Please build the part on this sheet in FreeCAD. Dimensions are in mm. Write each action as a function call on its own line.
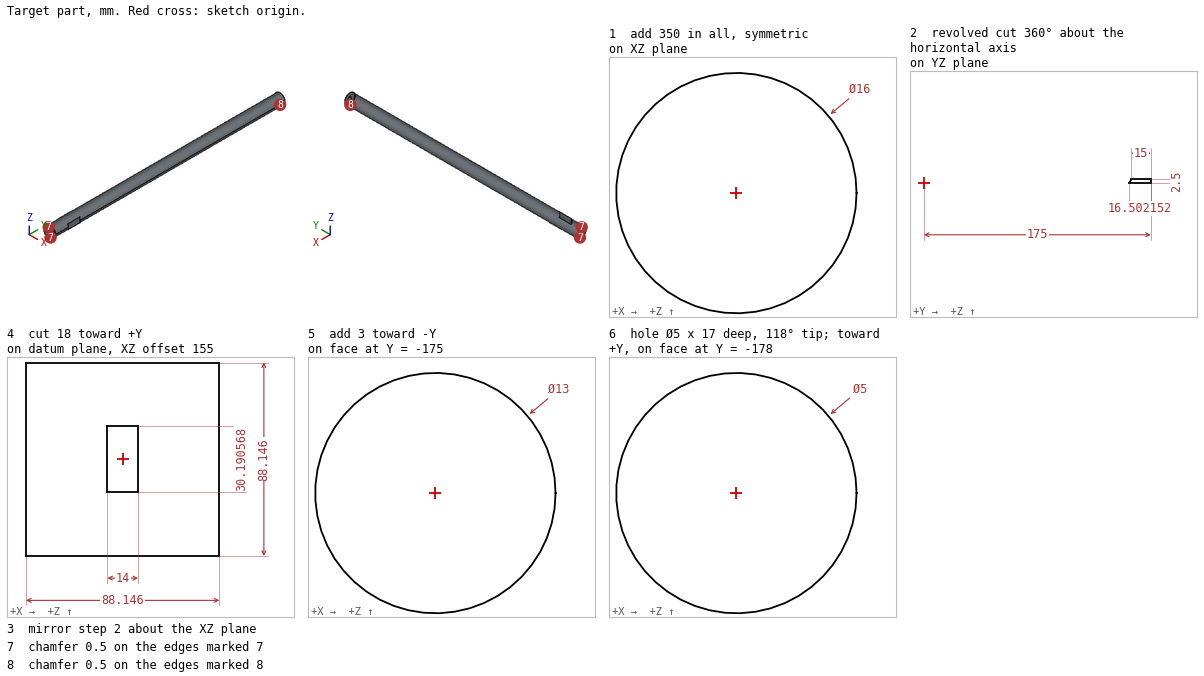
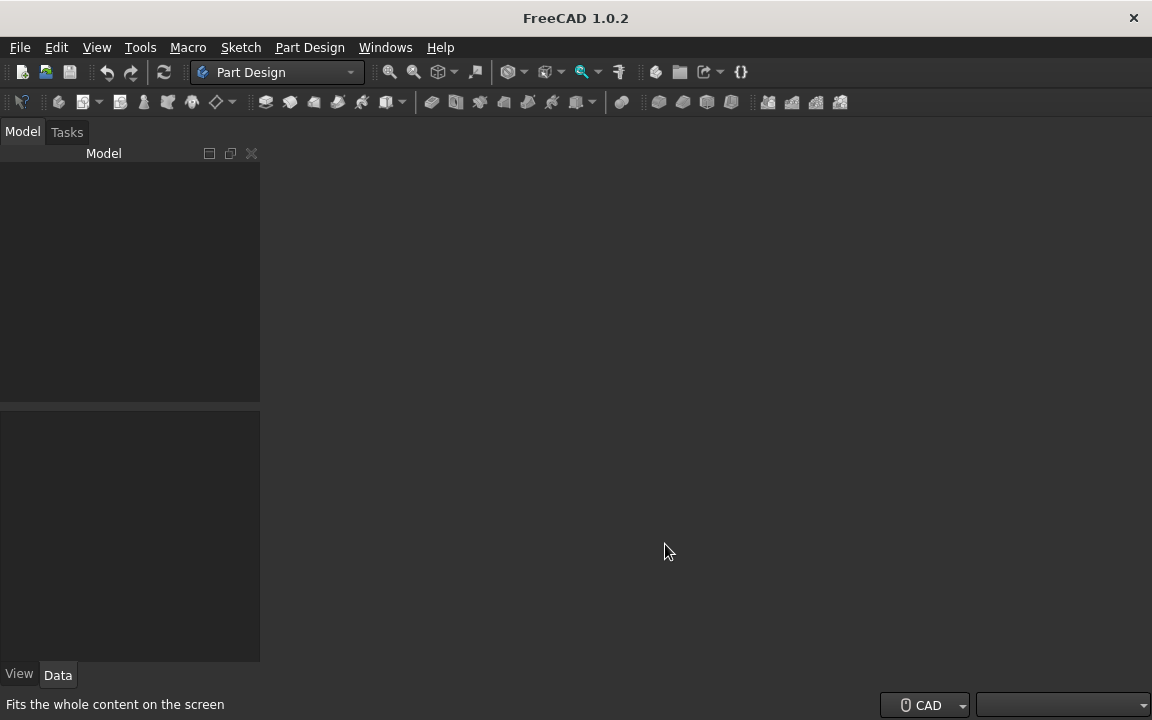
click(22, 72)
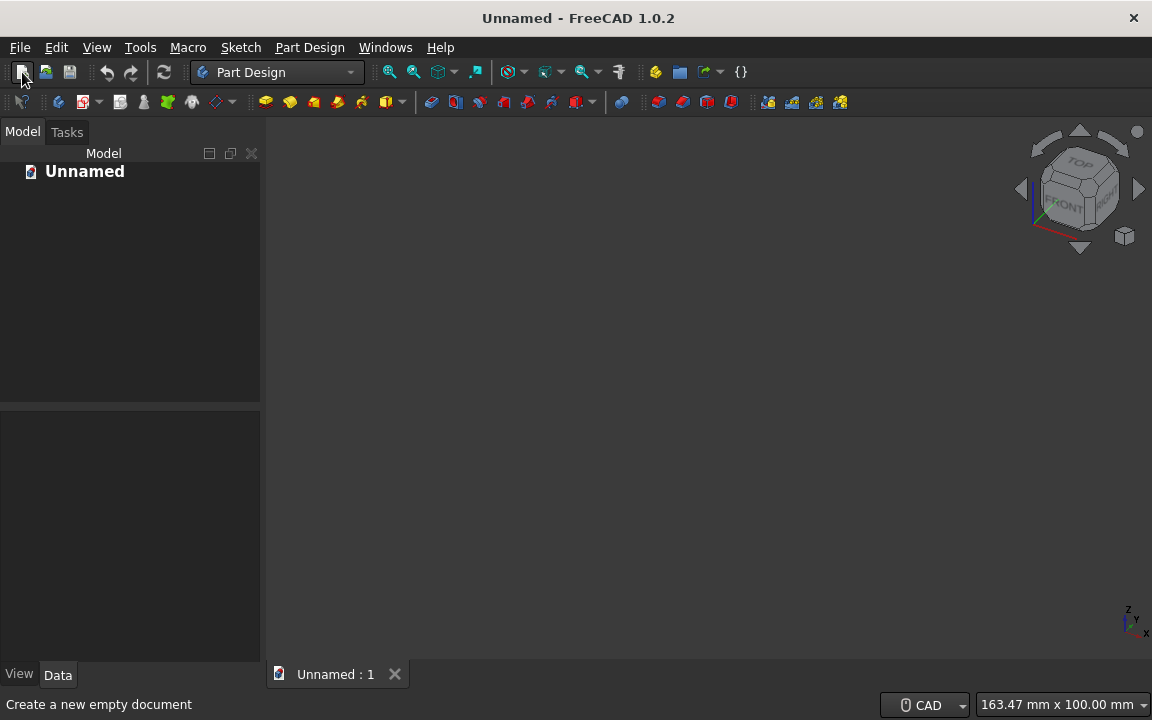
click(84, 102)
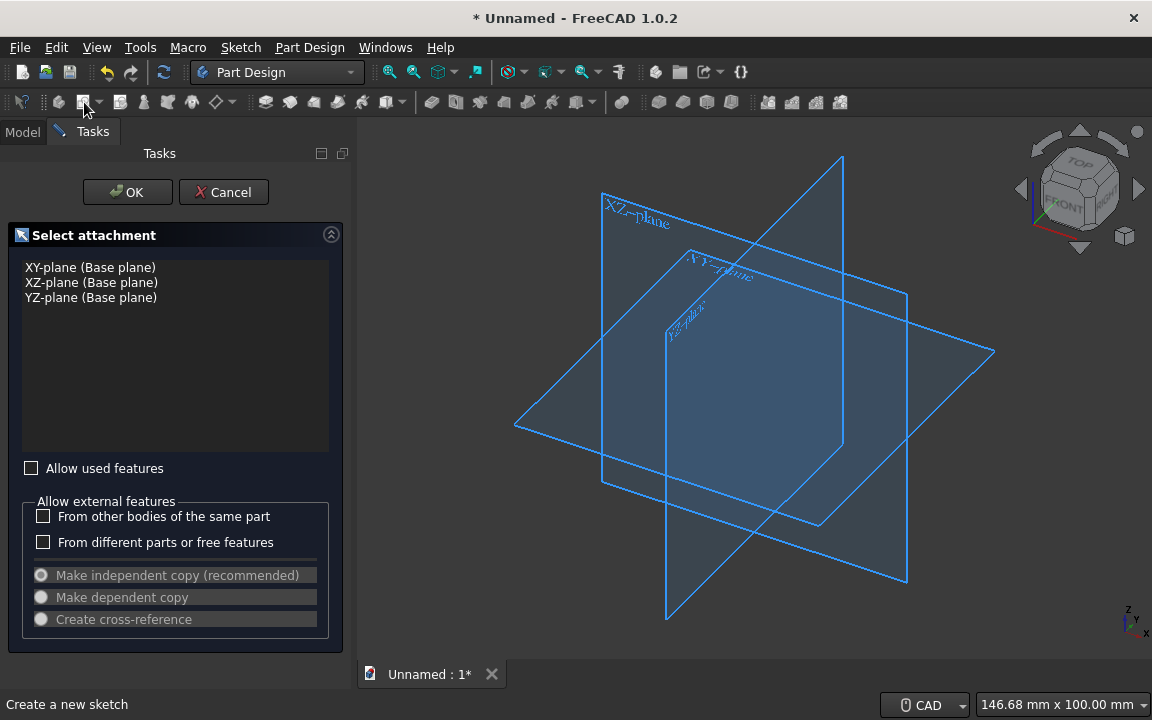
click(82, 282)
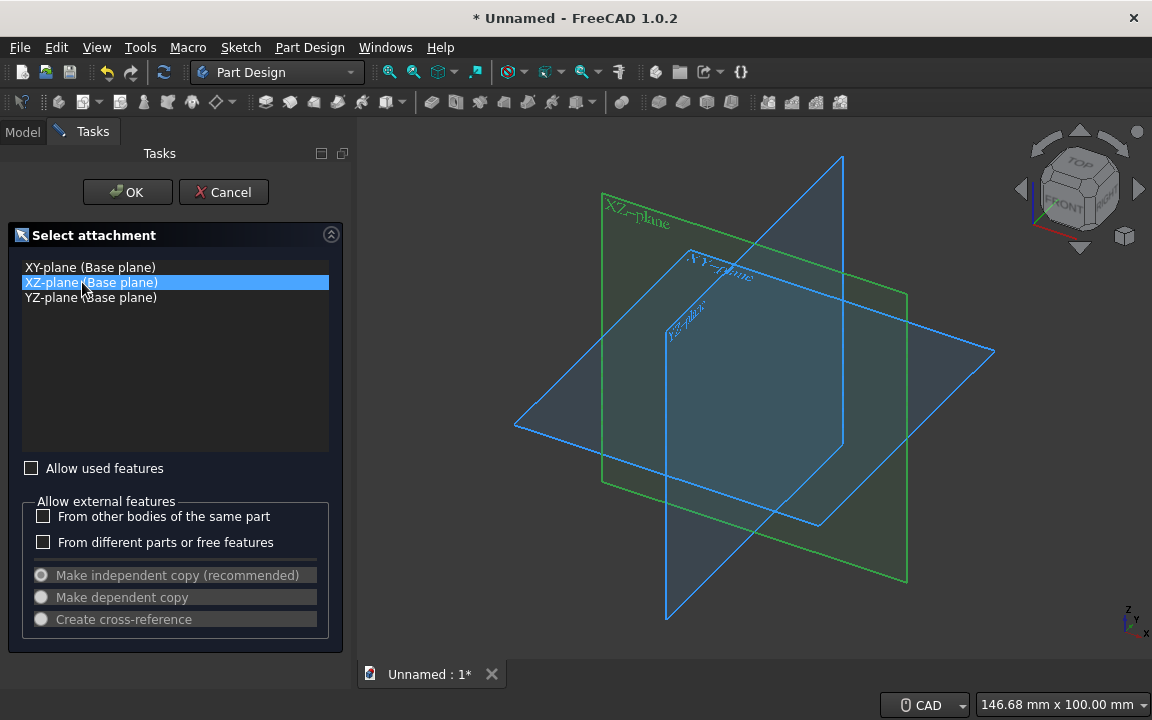
click(128, 192)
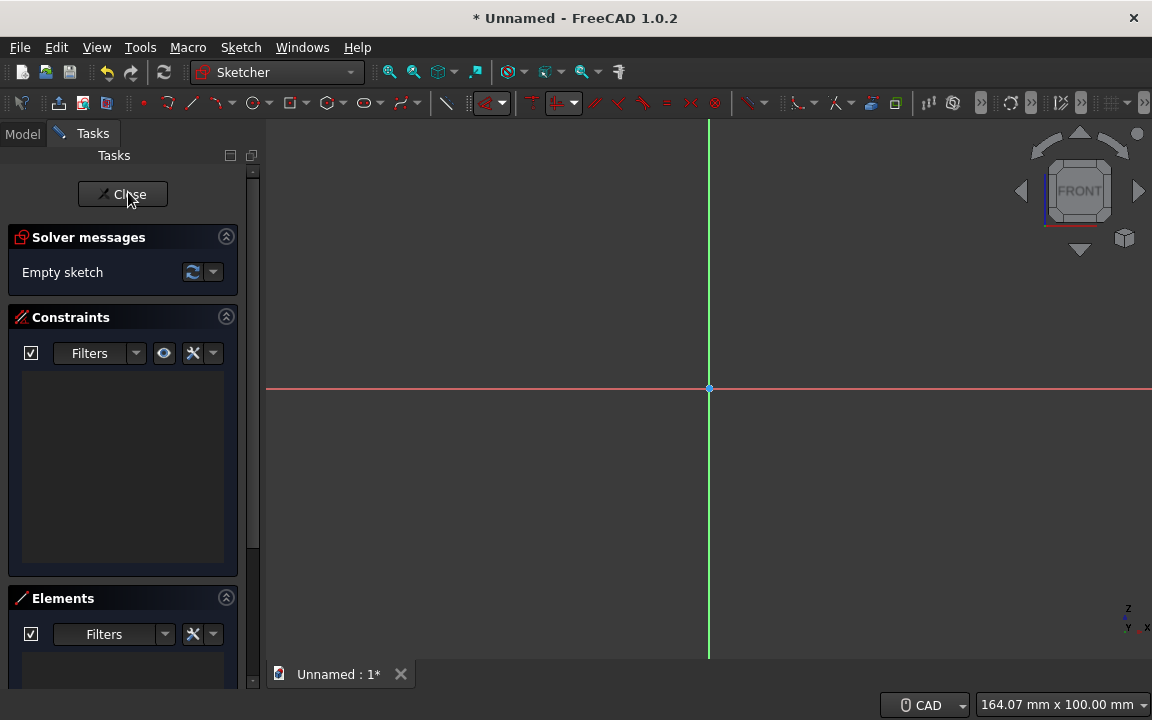
scroll(731, 389, up, 7)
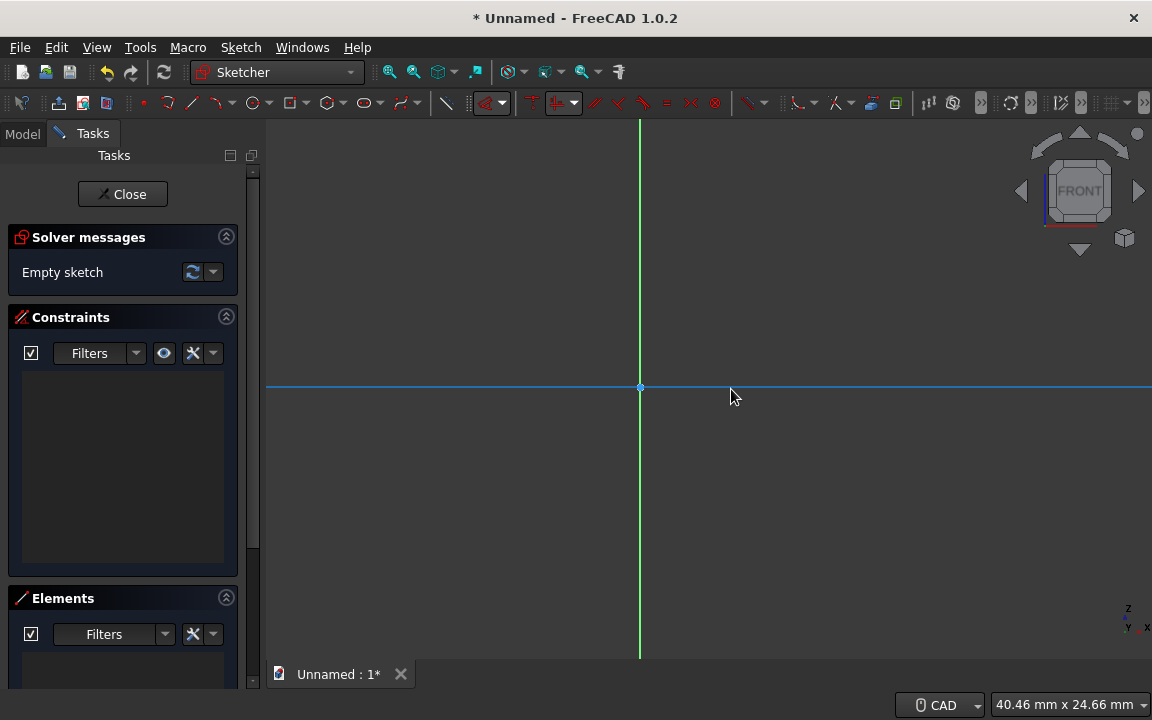
click(254, 104)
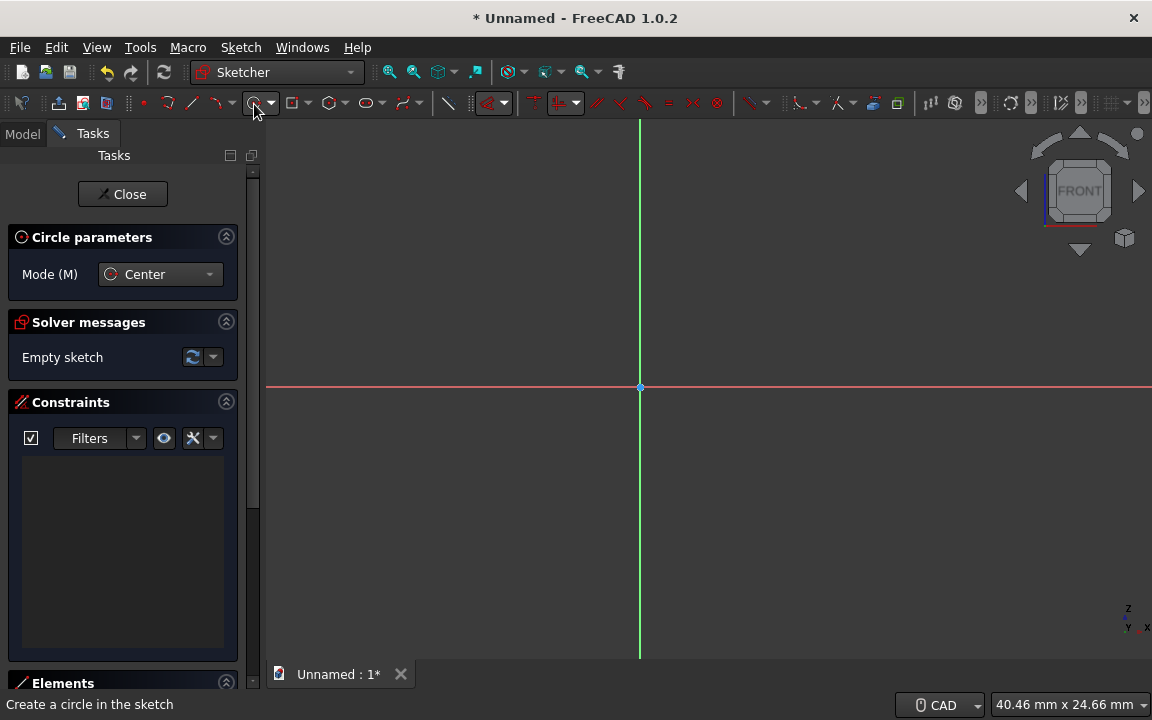
click(640, 387)
move(764, 264)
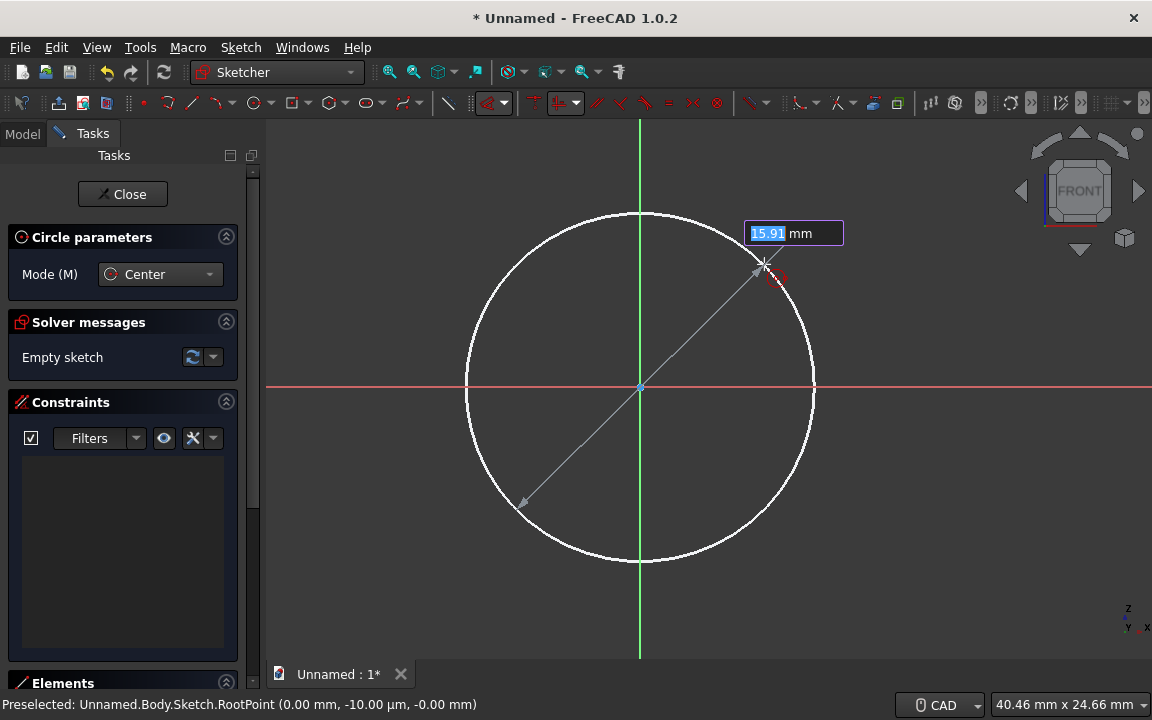
text(16)
key(Return)
key(Escape)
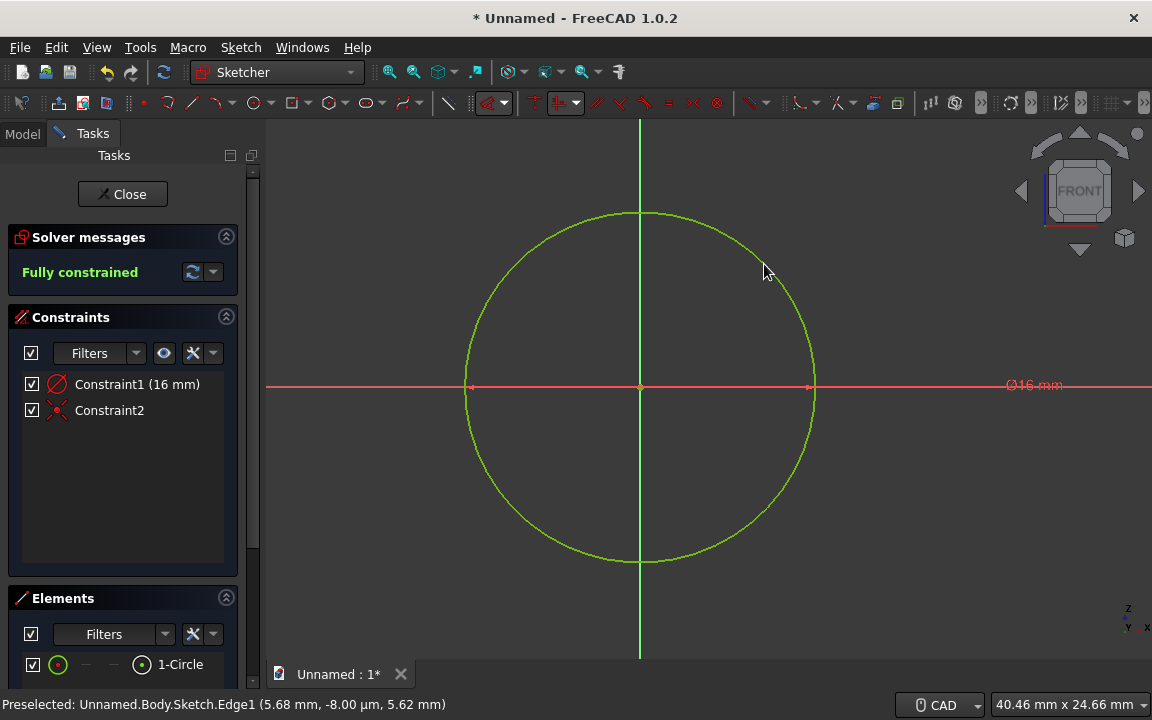
click(123, 194)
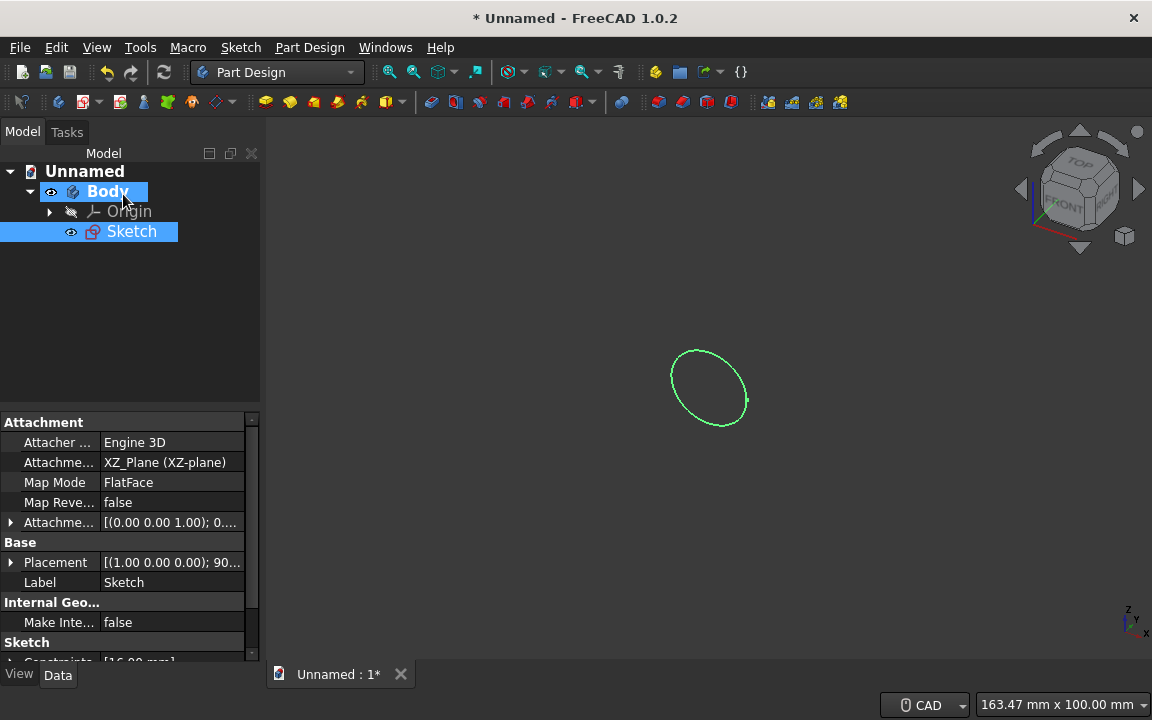
click(266, 102)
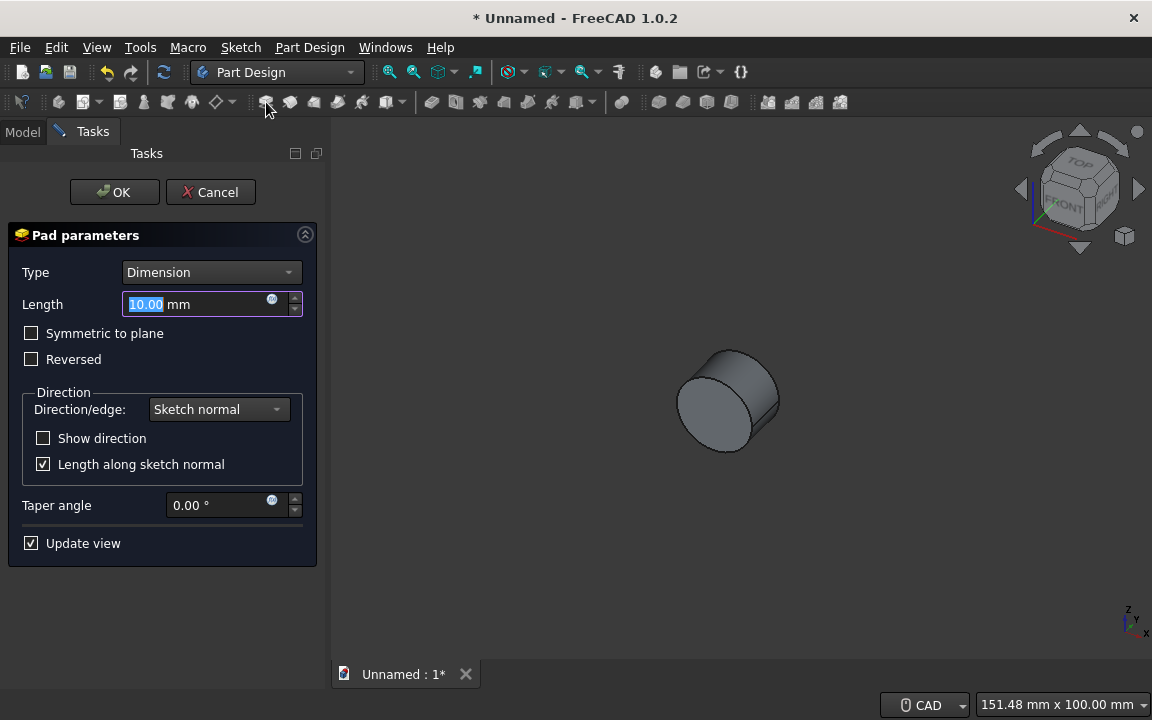
text(350)
key(Tab)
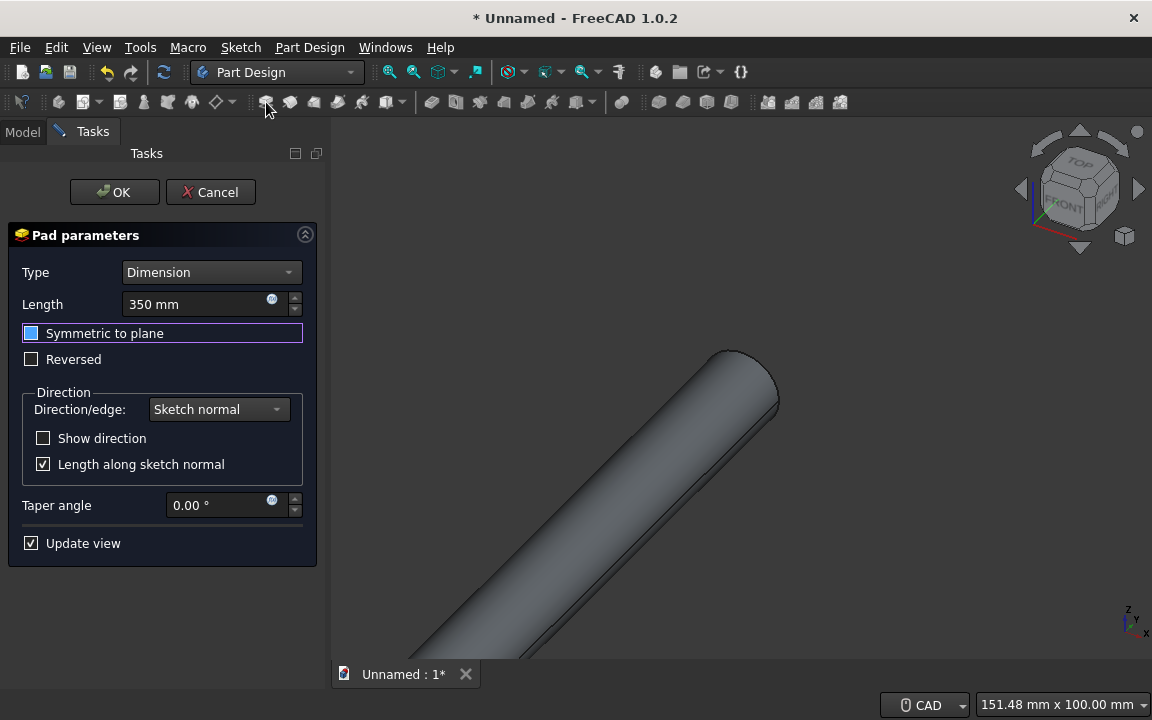
click(30, 333)